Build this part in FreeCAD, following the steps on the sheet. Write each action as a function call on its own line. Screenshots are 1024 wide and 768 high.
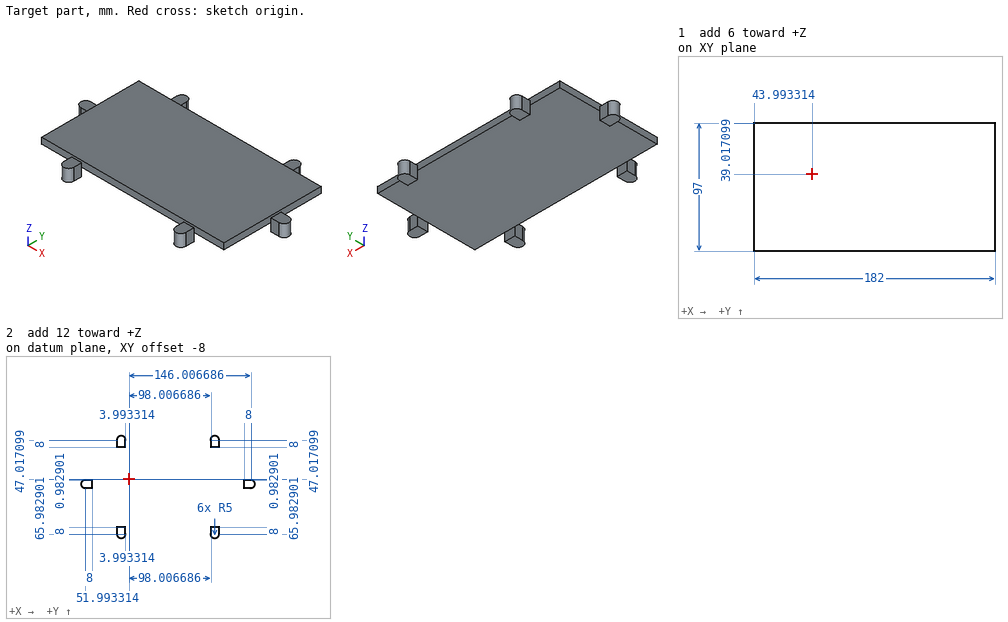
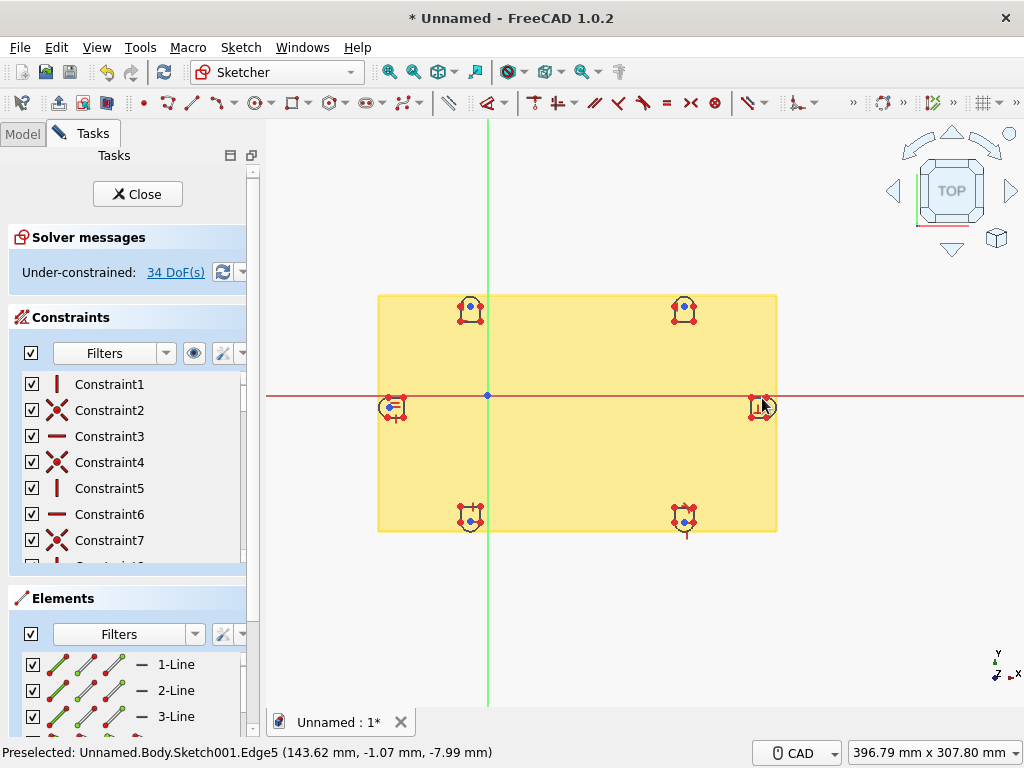
scroll(774, 413, up, 3)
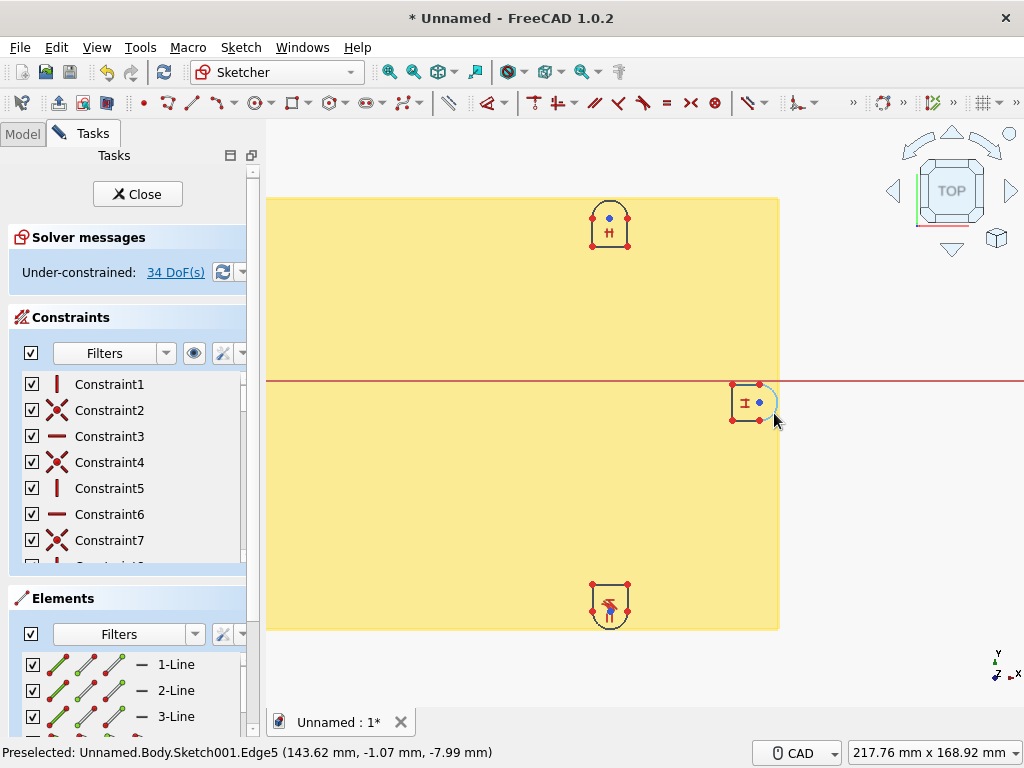
click(774, 413)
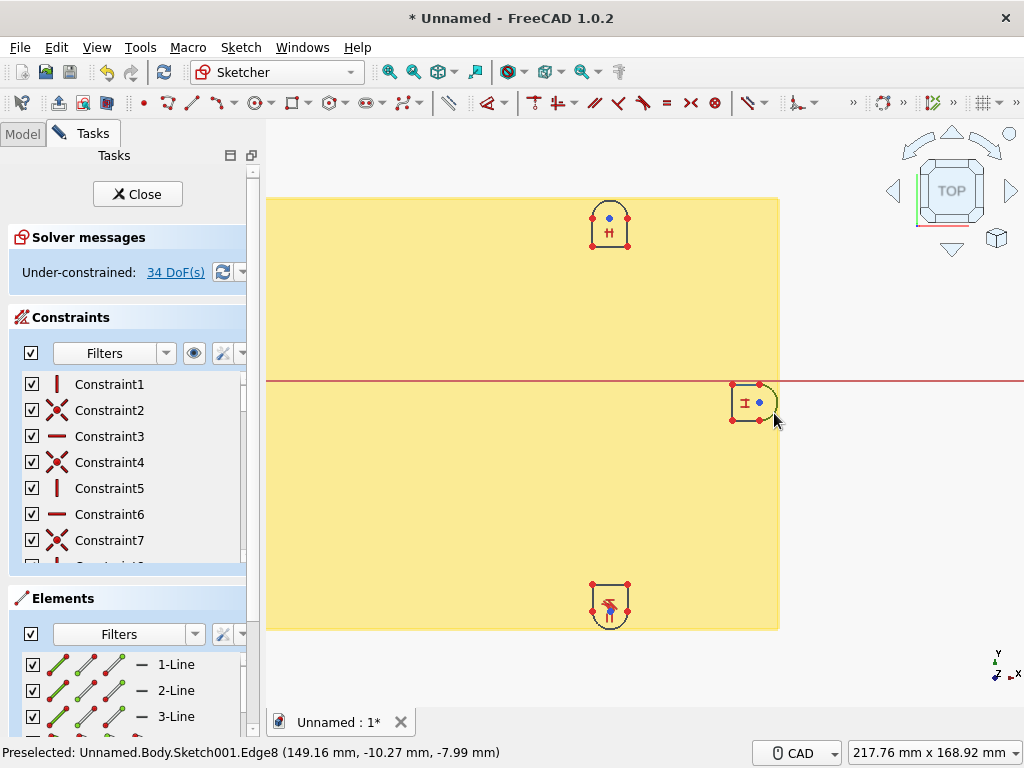
click(644, 104)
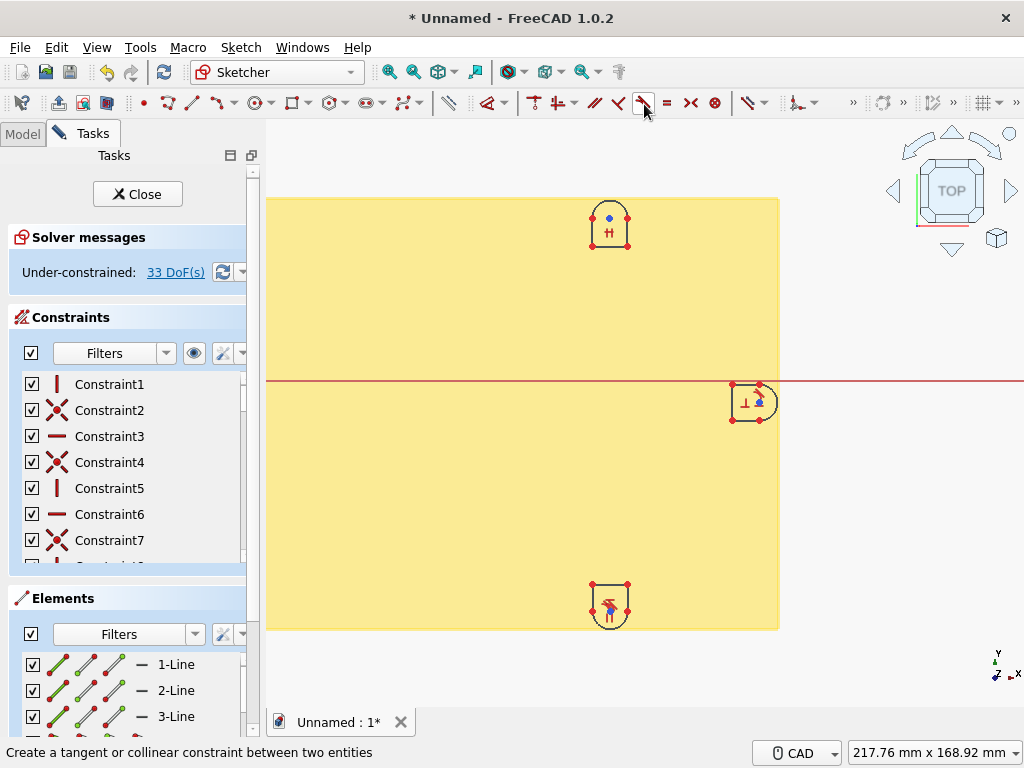
scroll(743, 421, up, 2)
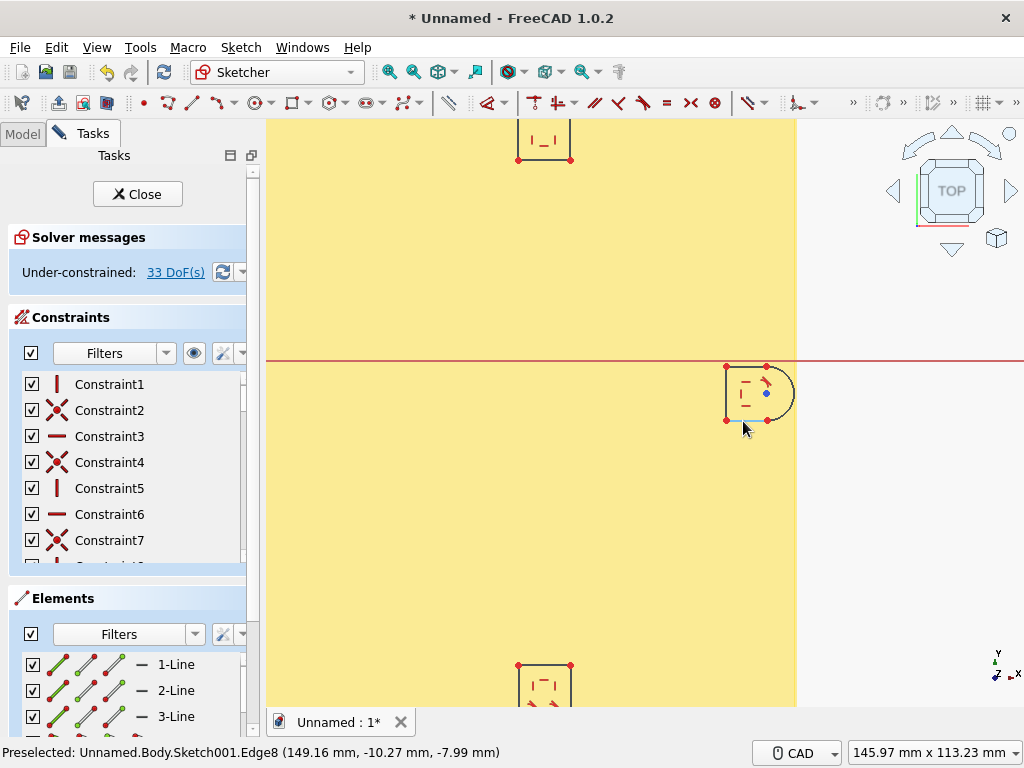
click(743, 421)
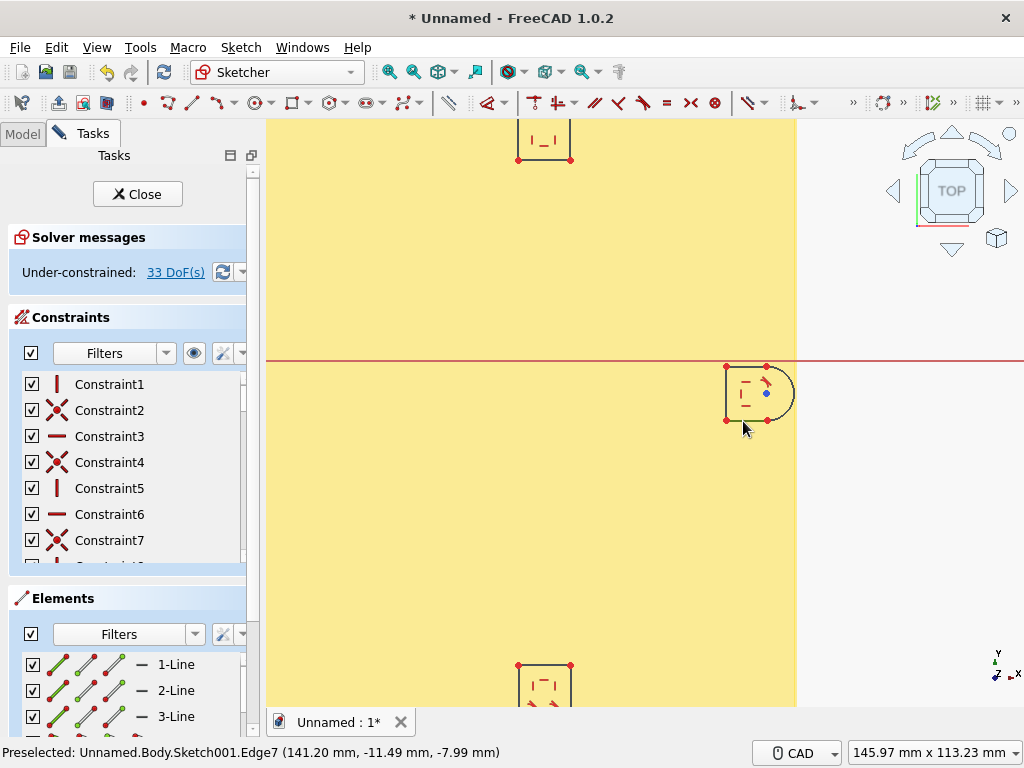
click(789, 409)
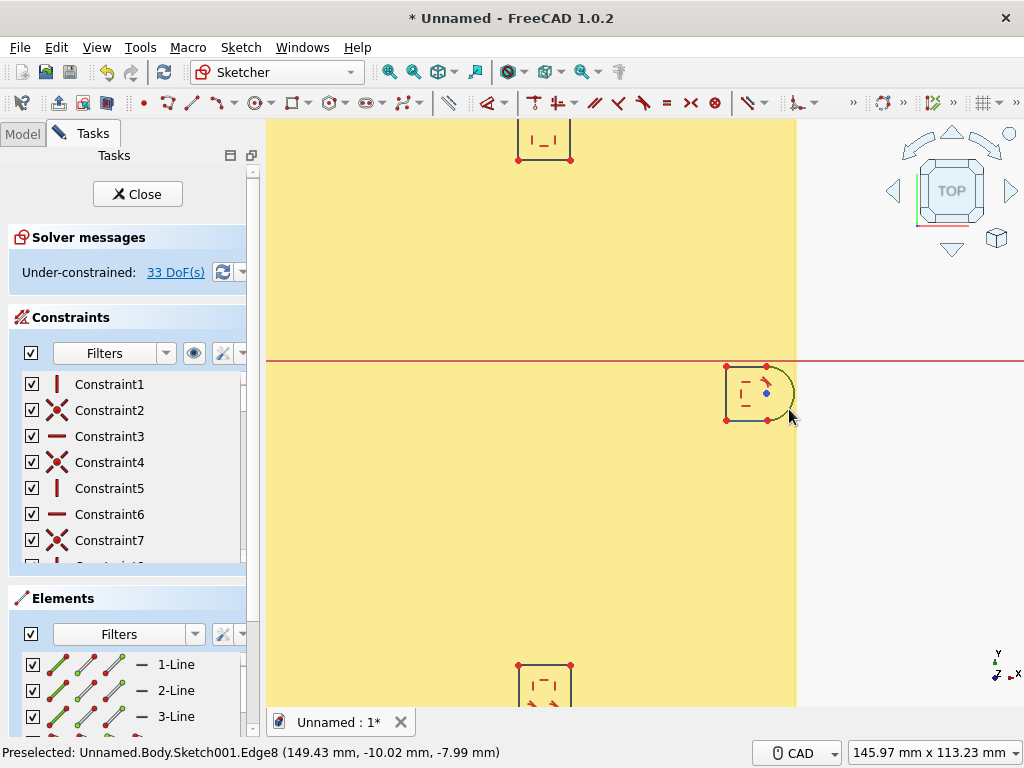
click(644, 104)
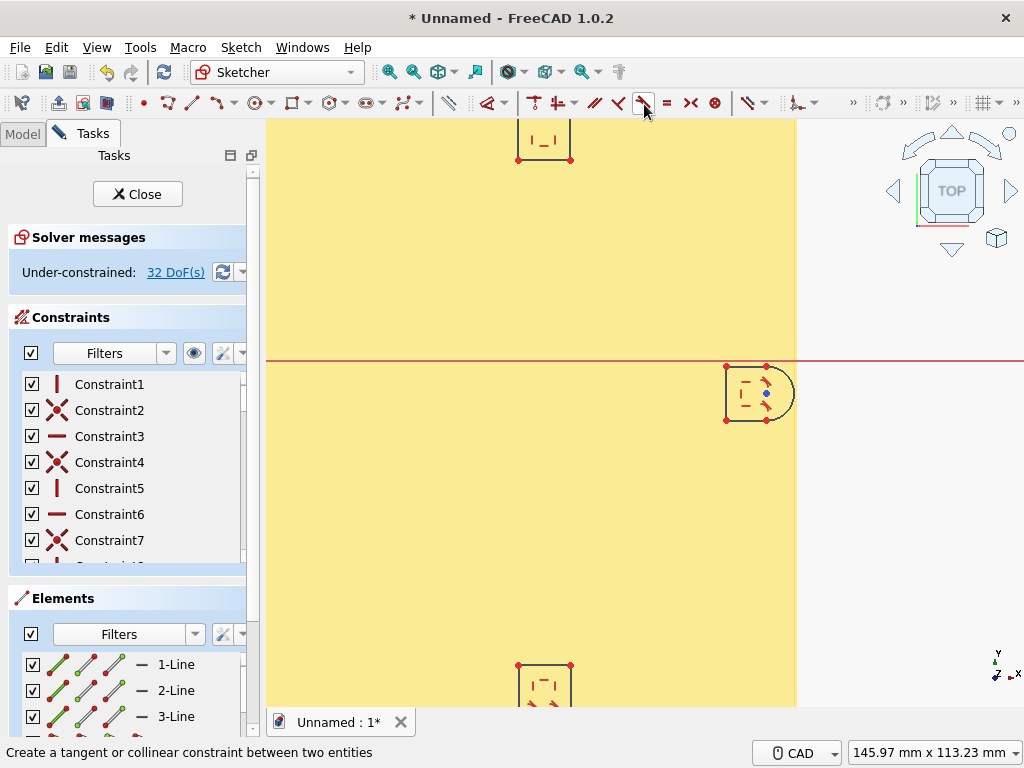
click(518, 148)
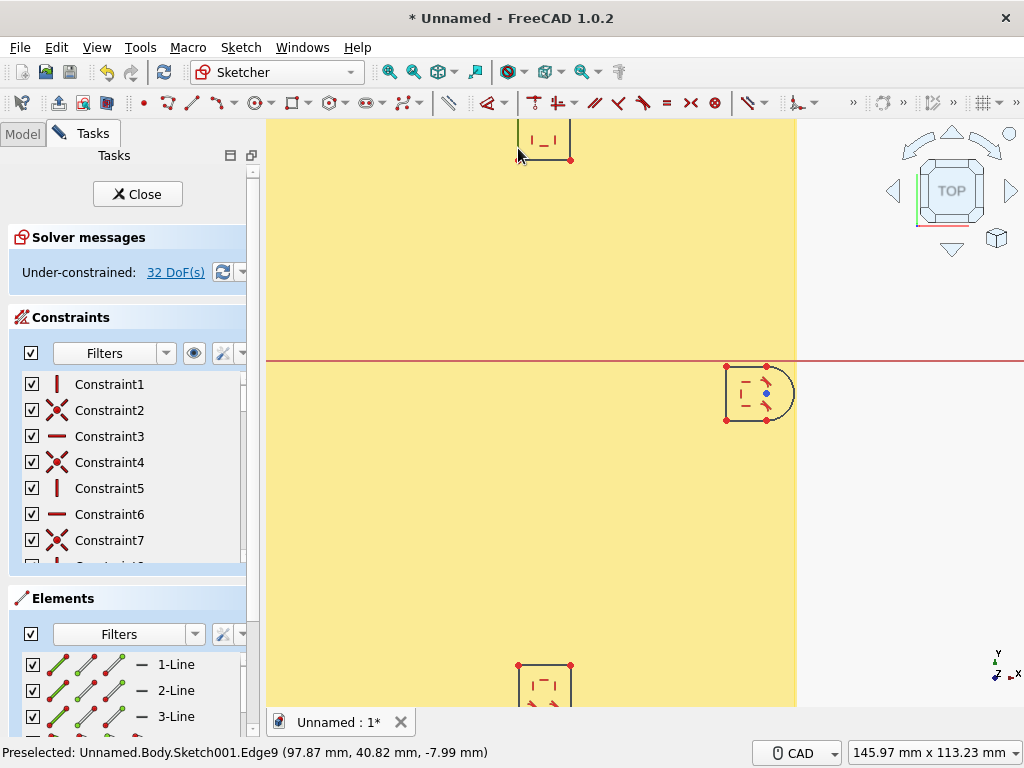
scroll(764, 415, down, 5)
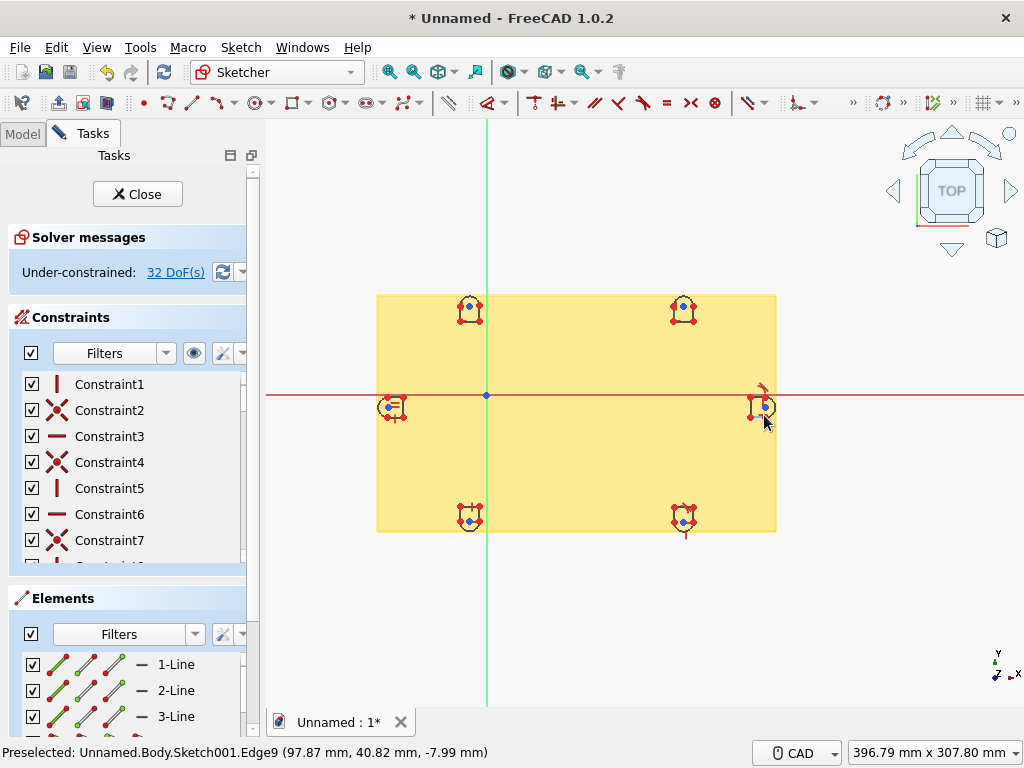
scroll(689, 298, up, 3)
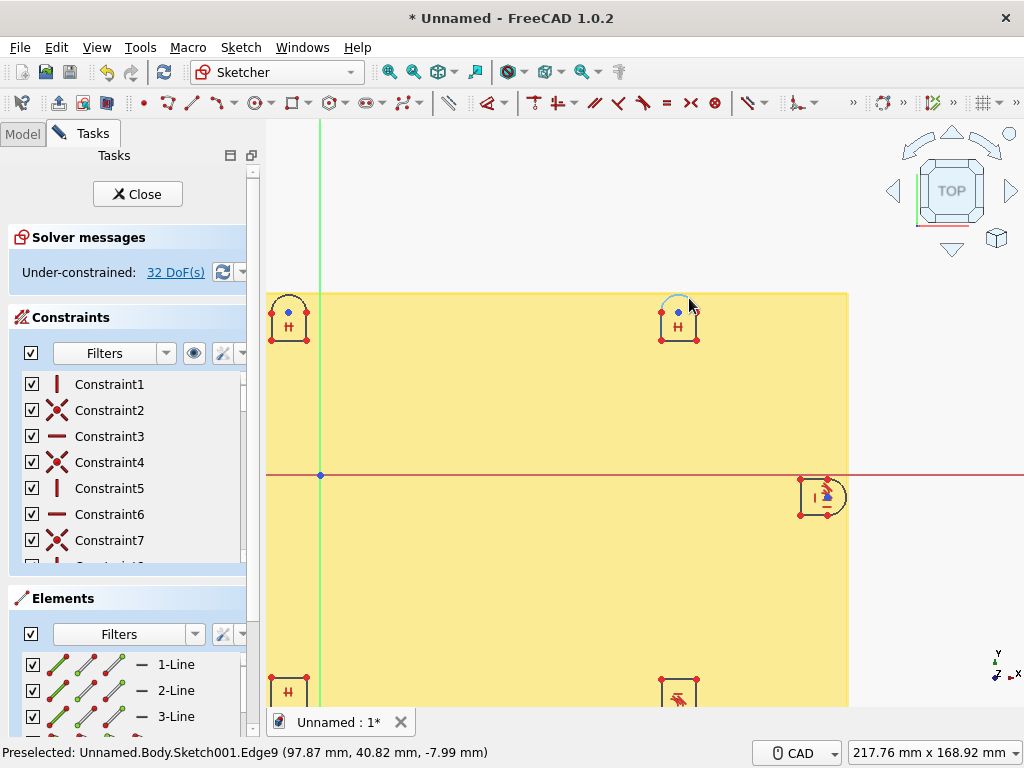
click(689, 298)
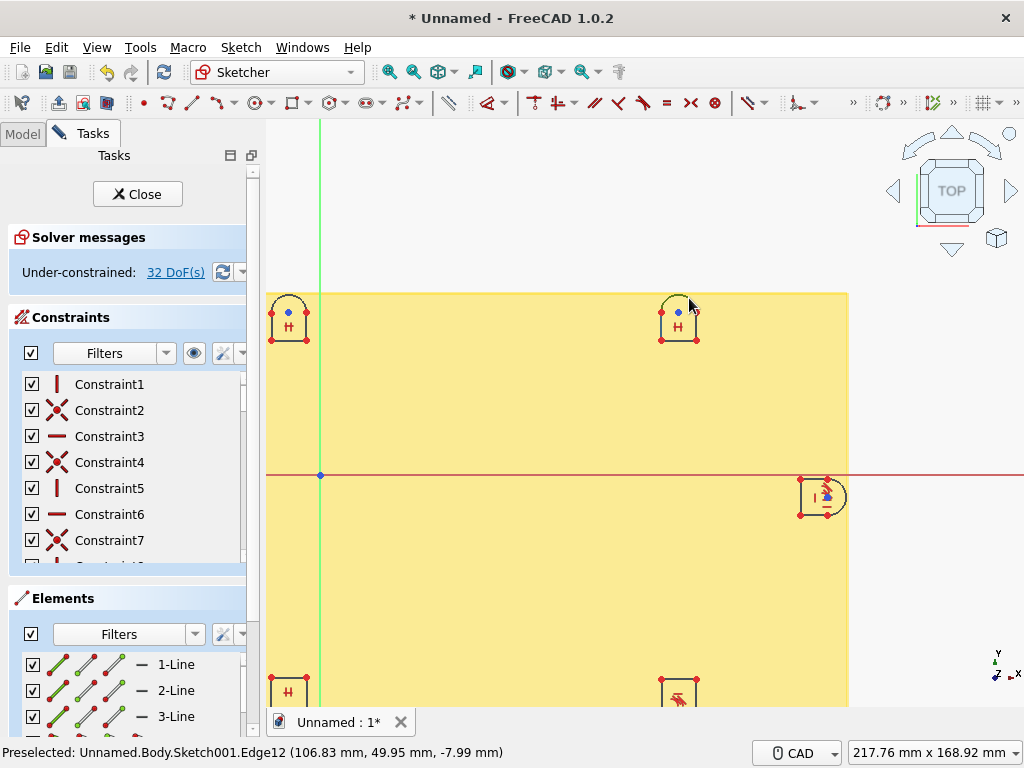
click(644, 104)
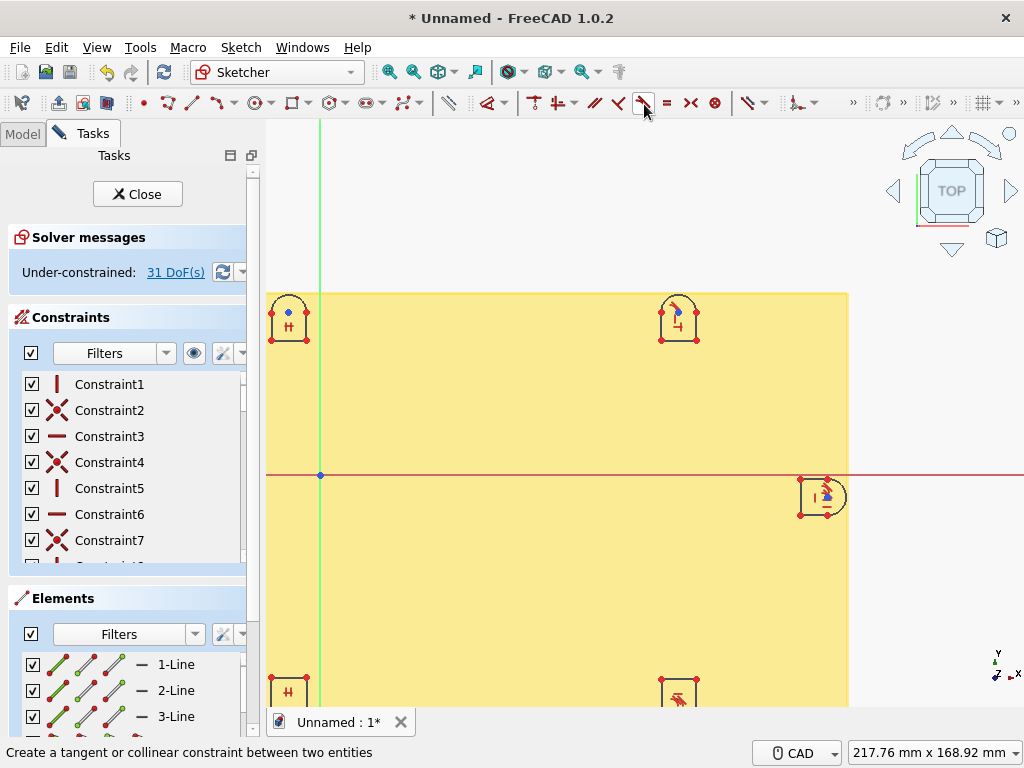
scroll(696, 330, up, 2)